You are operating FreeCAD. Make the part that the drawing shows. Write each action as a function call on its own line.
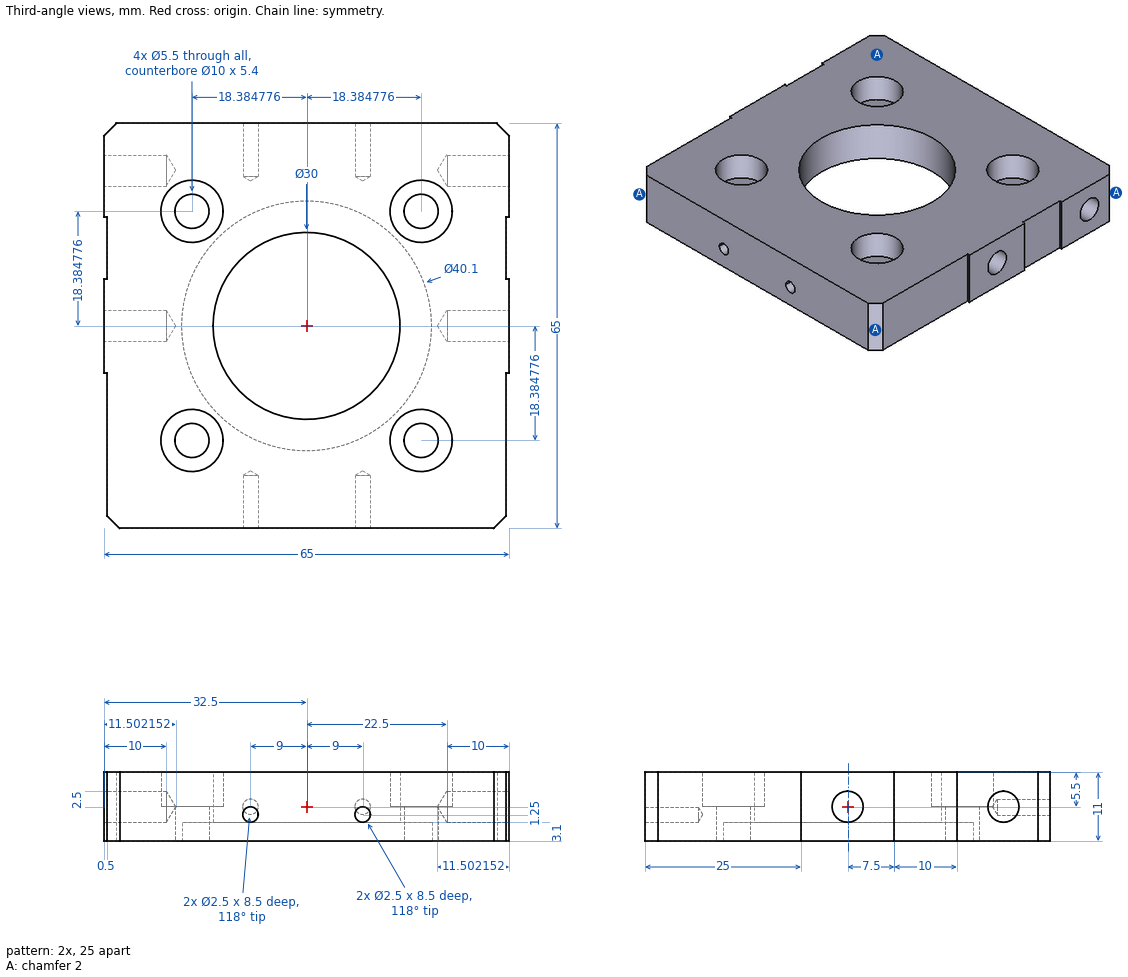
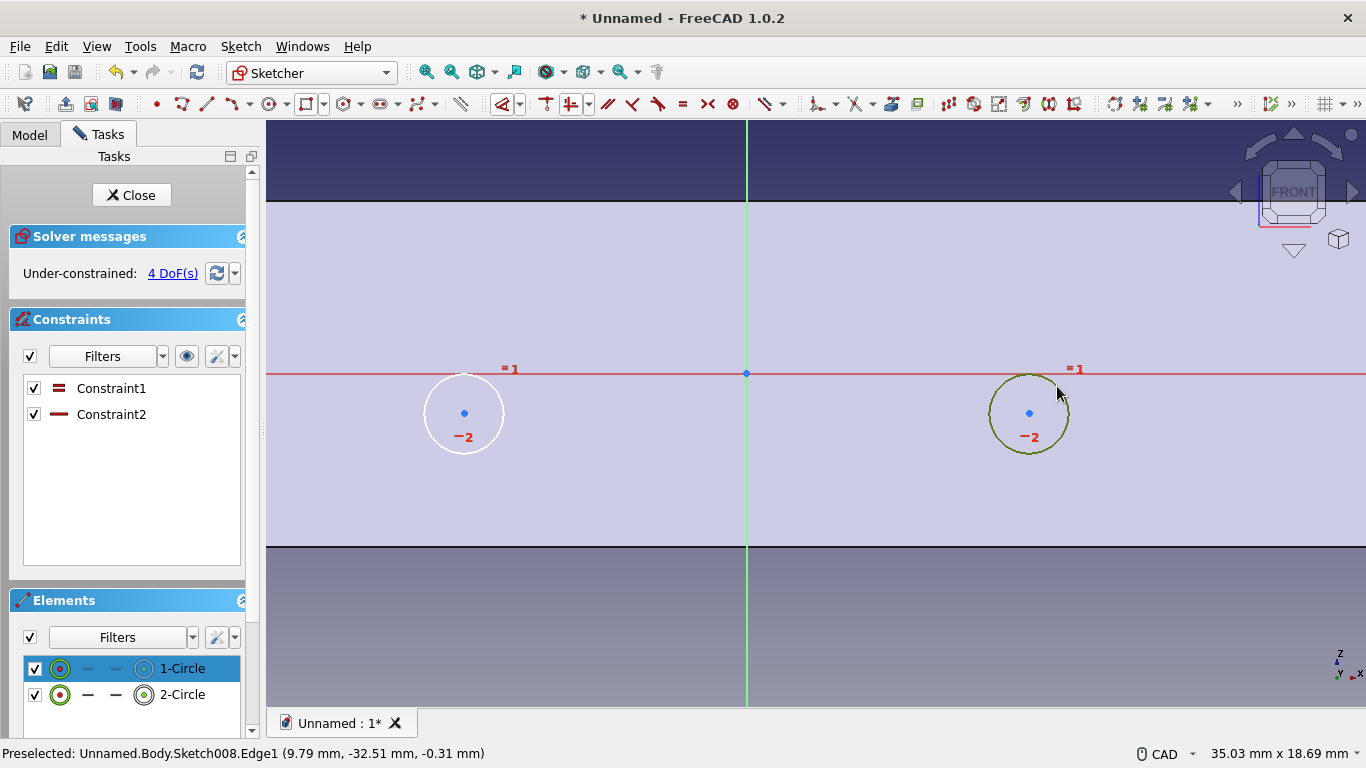
click(520, 104)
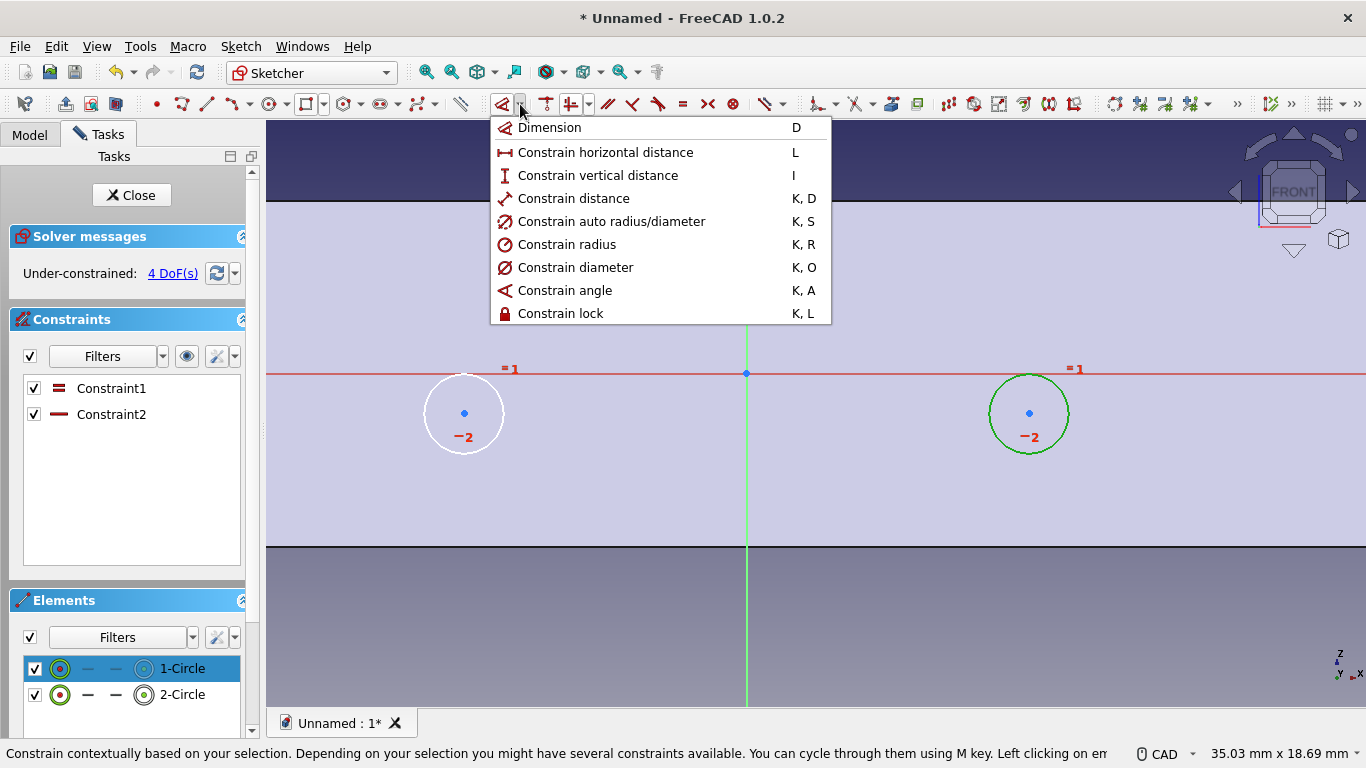
click(661, 268)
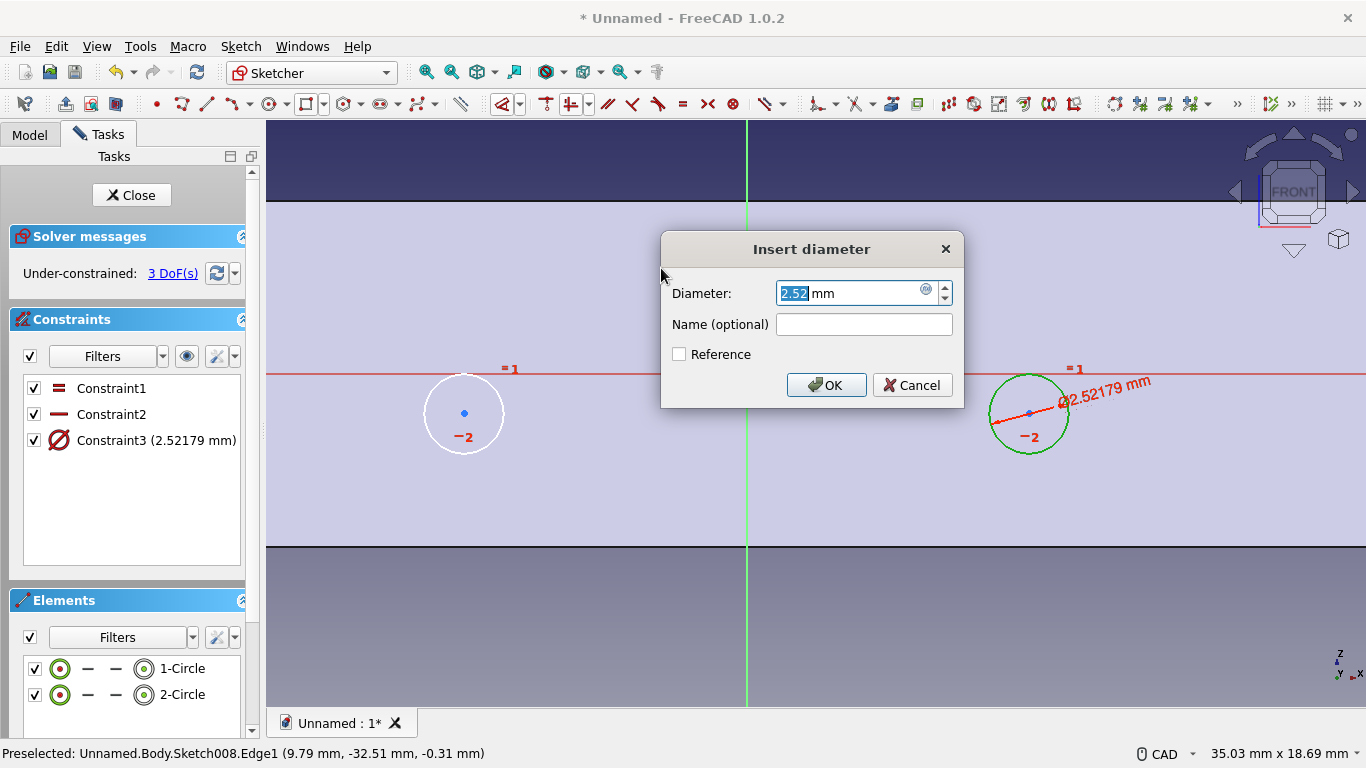
text(2.5)
key(Return)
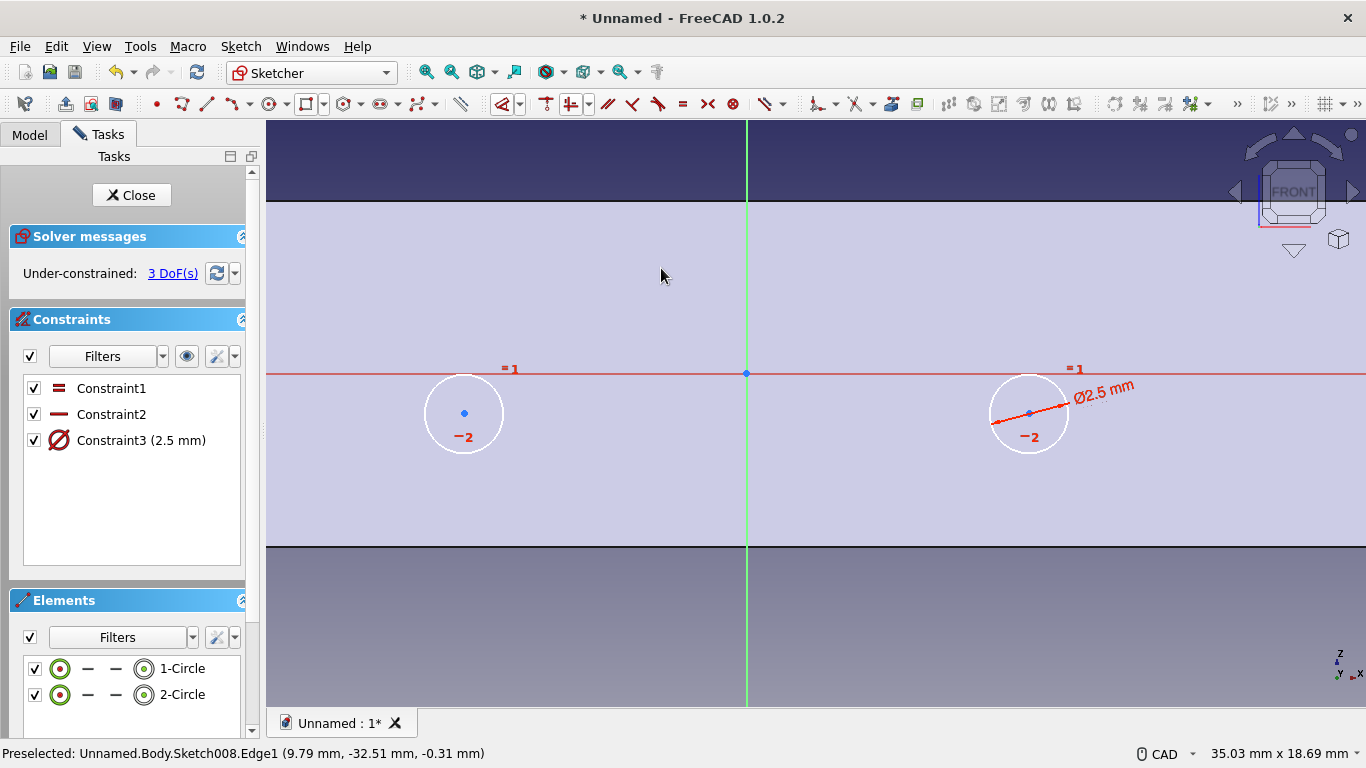
click(1029, 414)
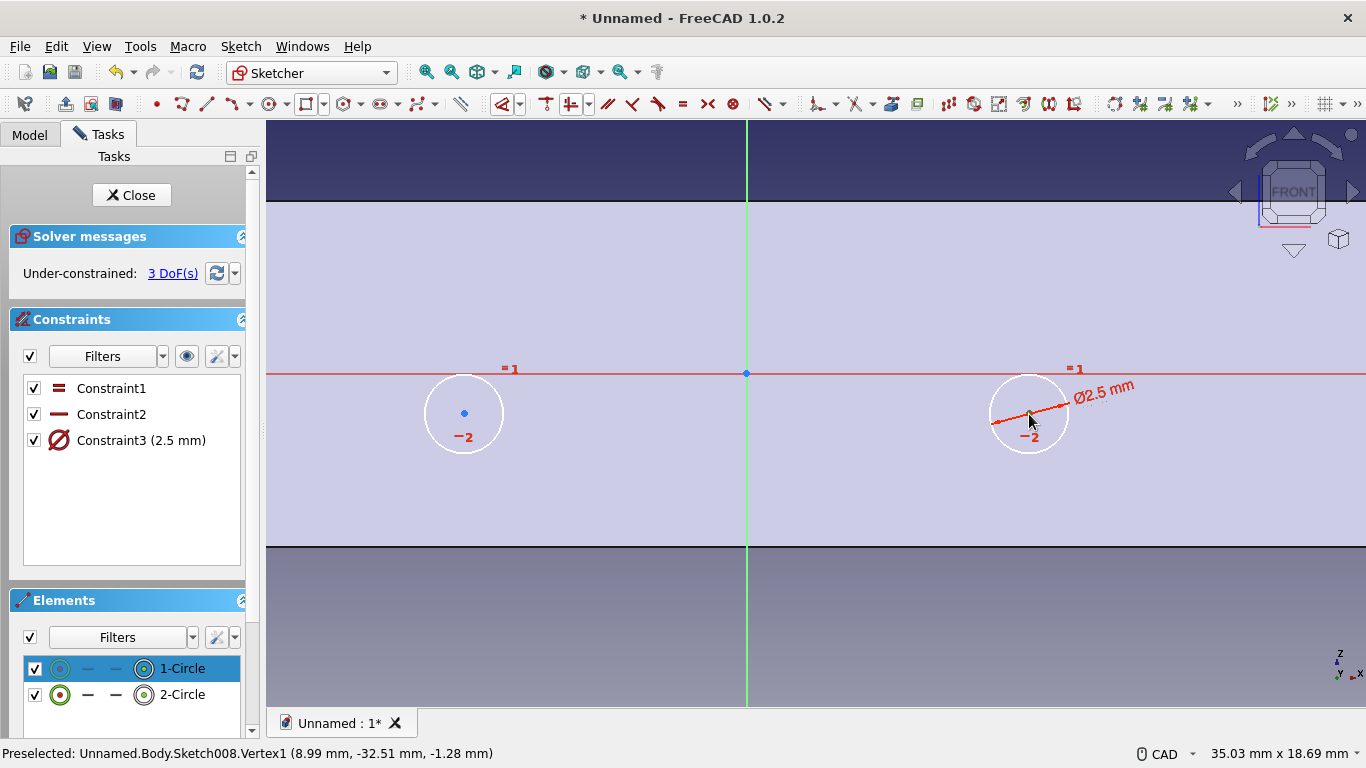
click(520, 104)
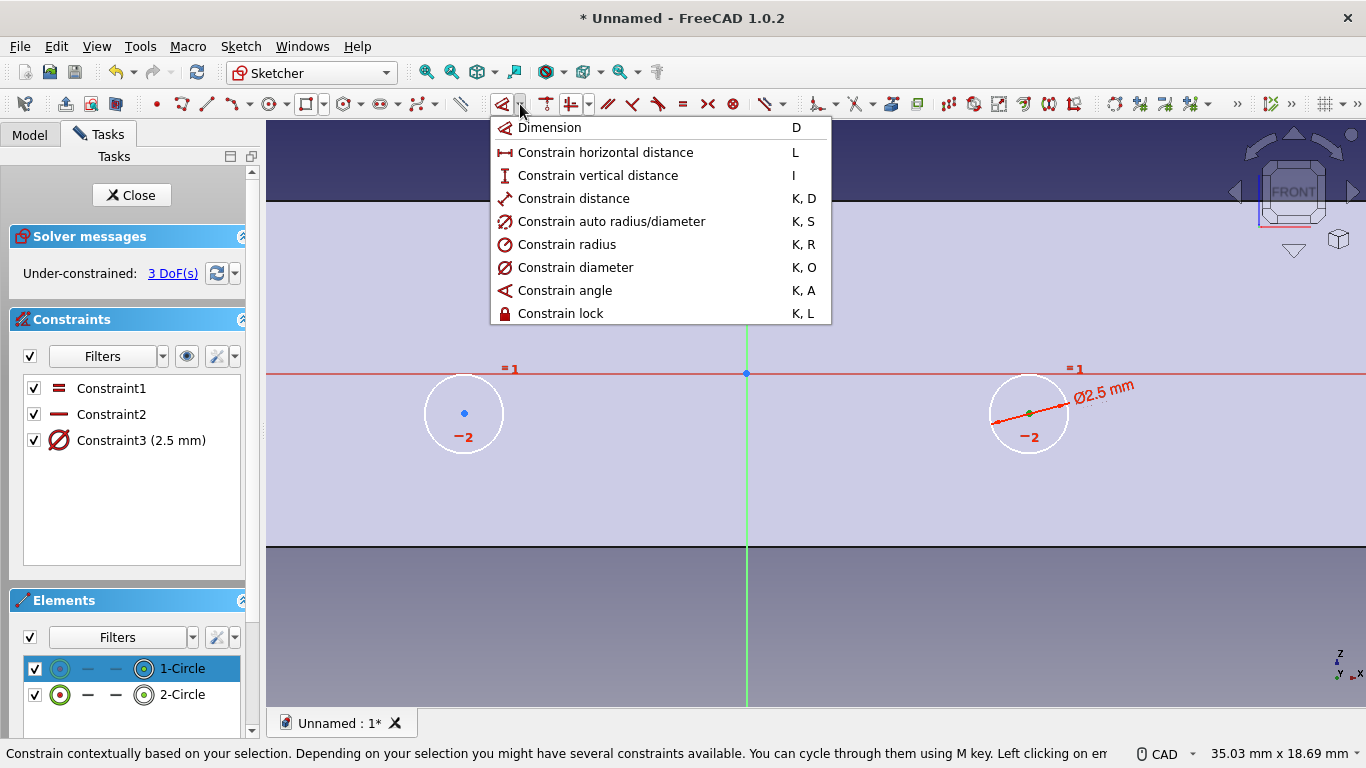
click(661, 152)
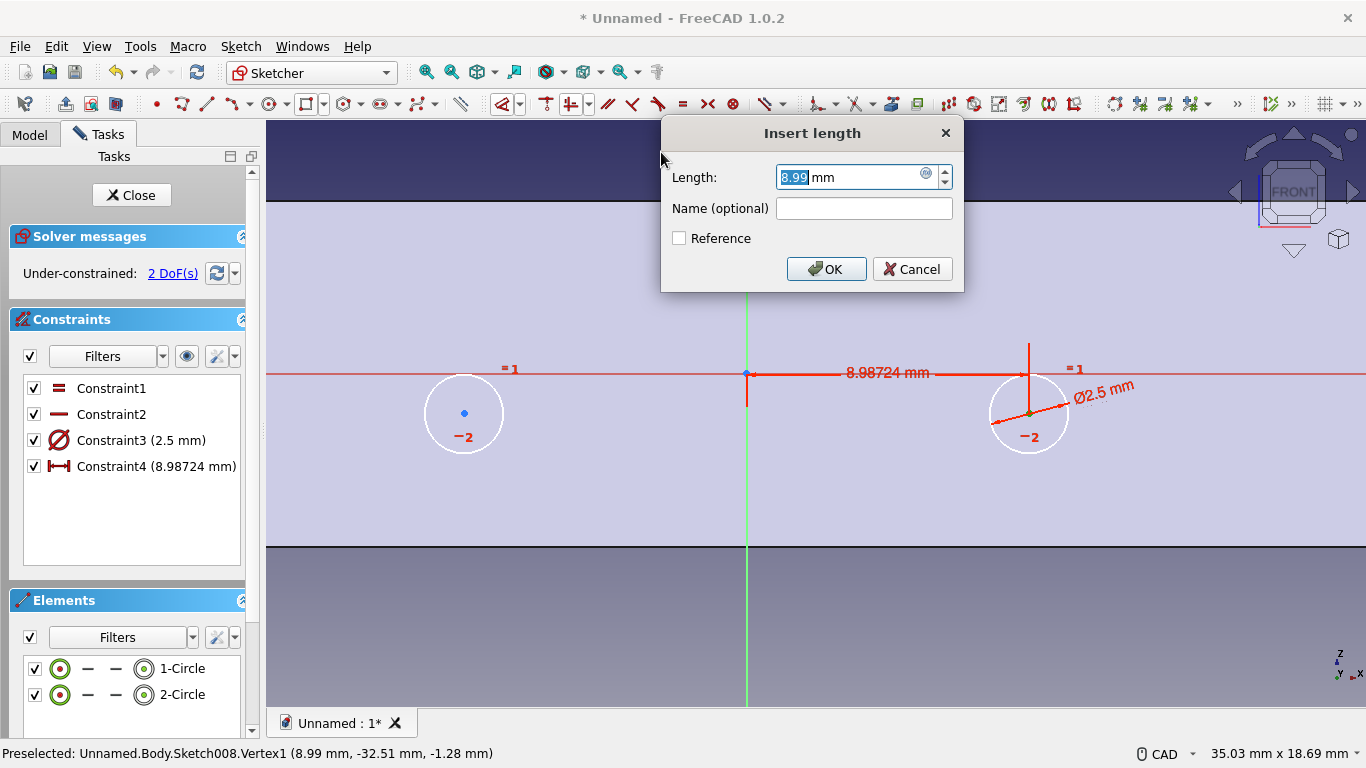
text(9)
key(Return)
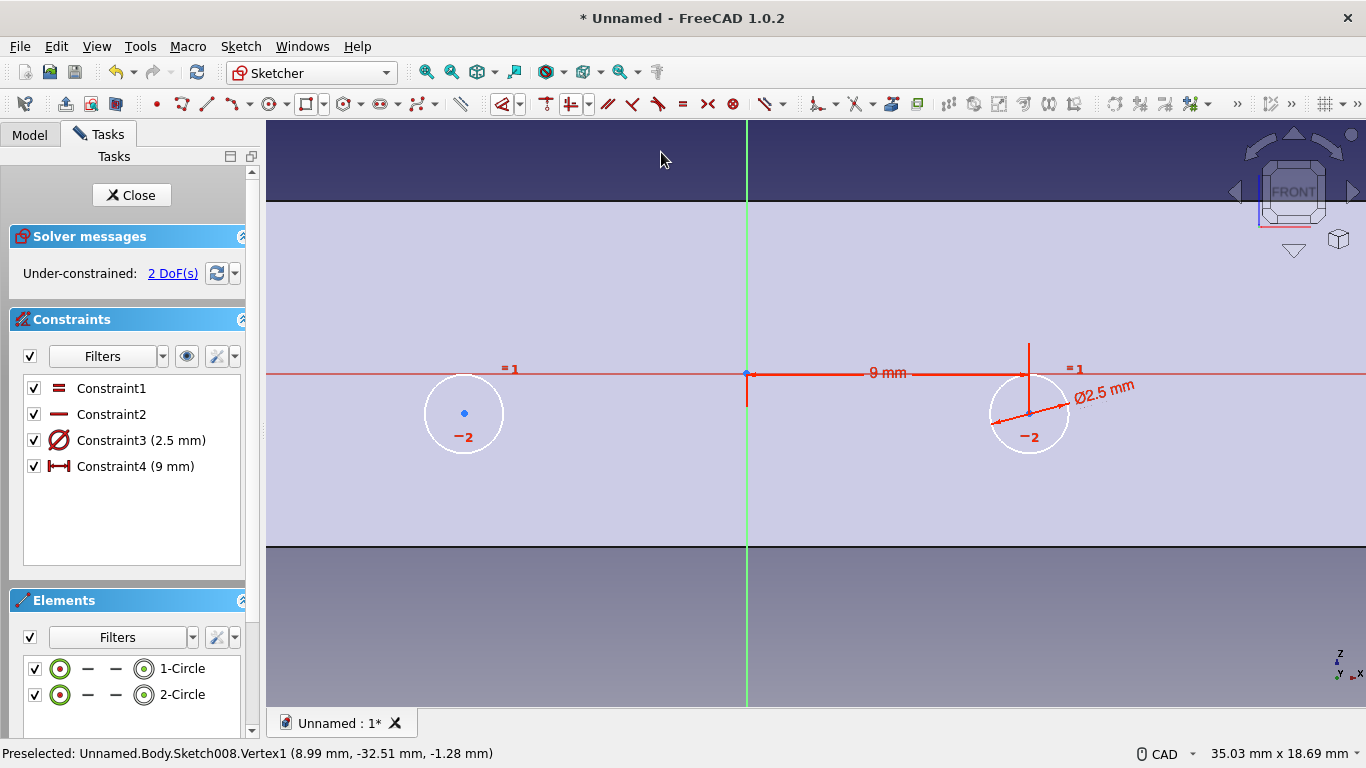
click(464, 414)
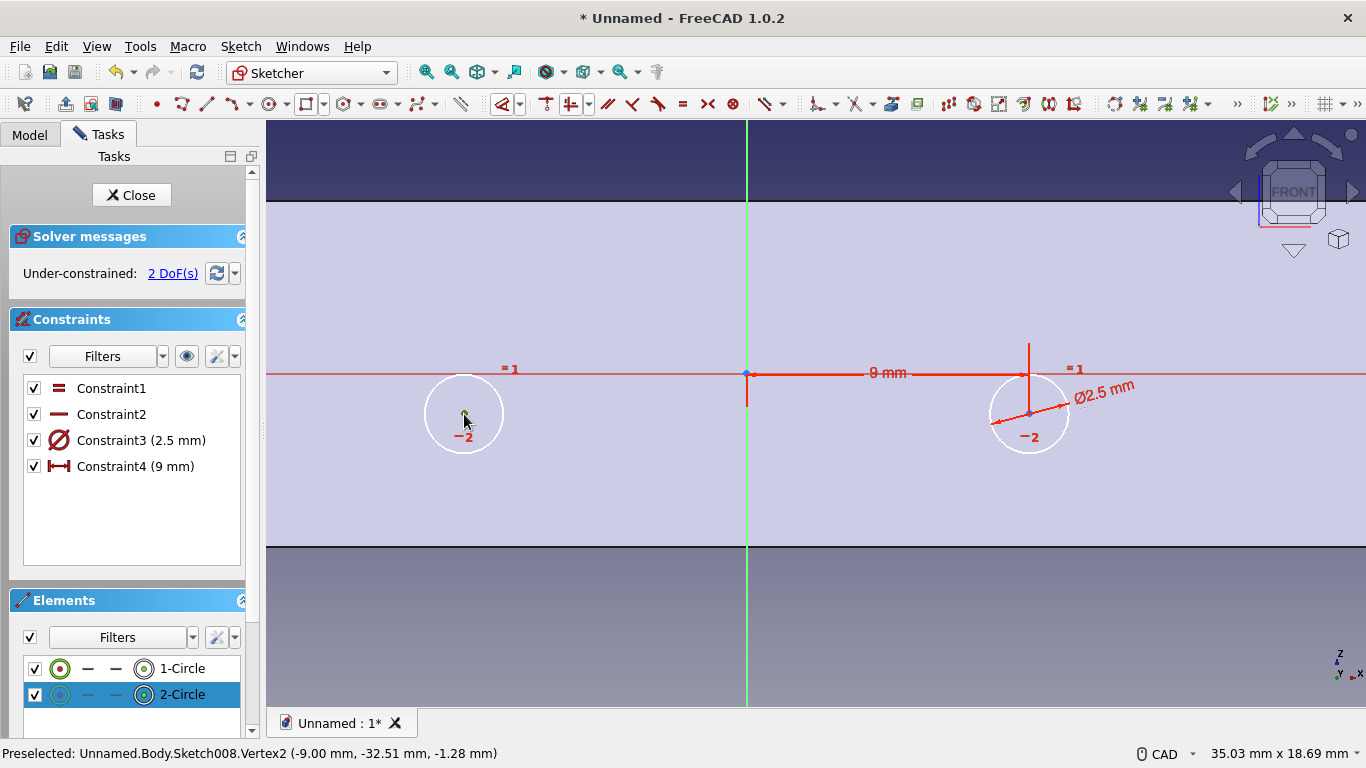
key(l)